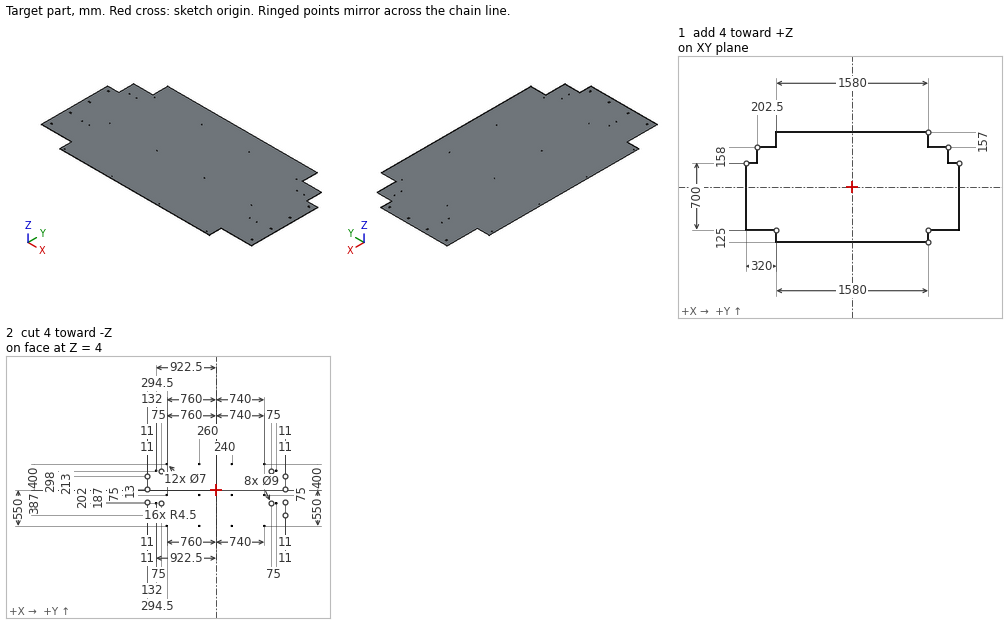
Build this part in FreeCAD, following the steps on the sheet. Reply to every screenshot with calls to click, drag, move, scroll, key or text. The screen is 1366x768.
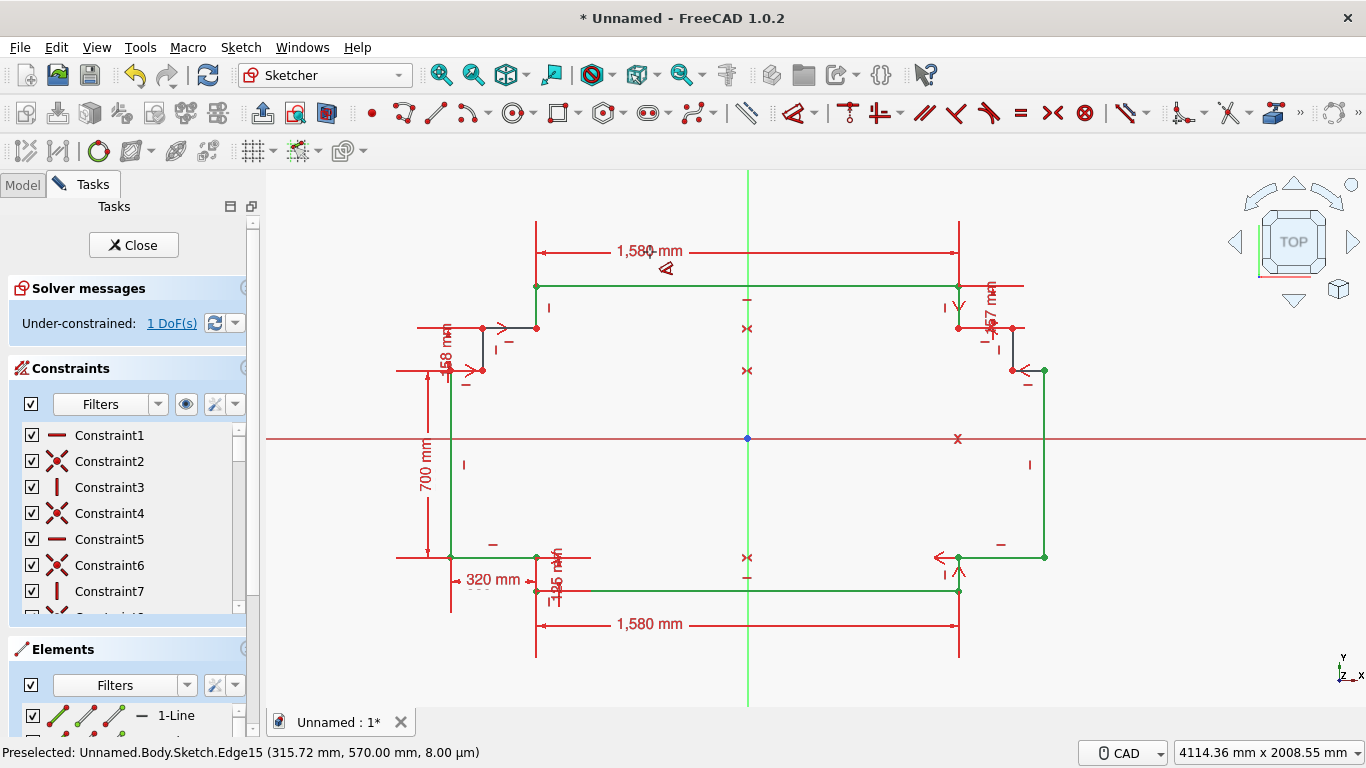
click(520, 328)
click(509, 294)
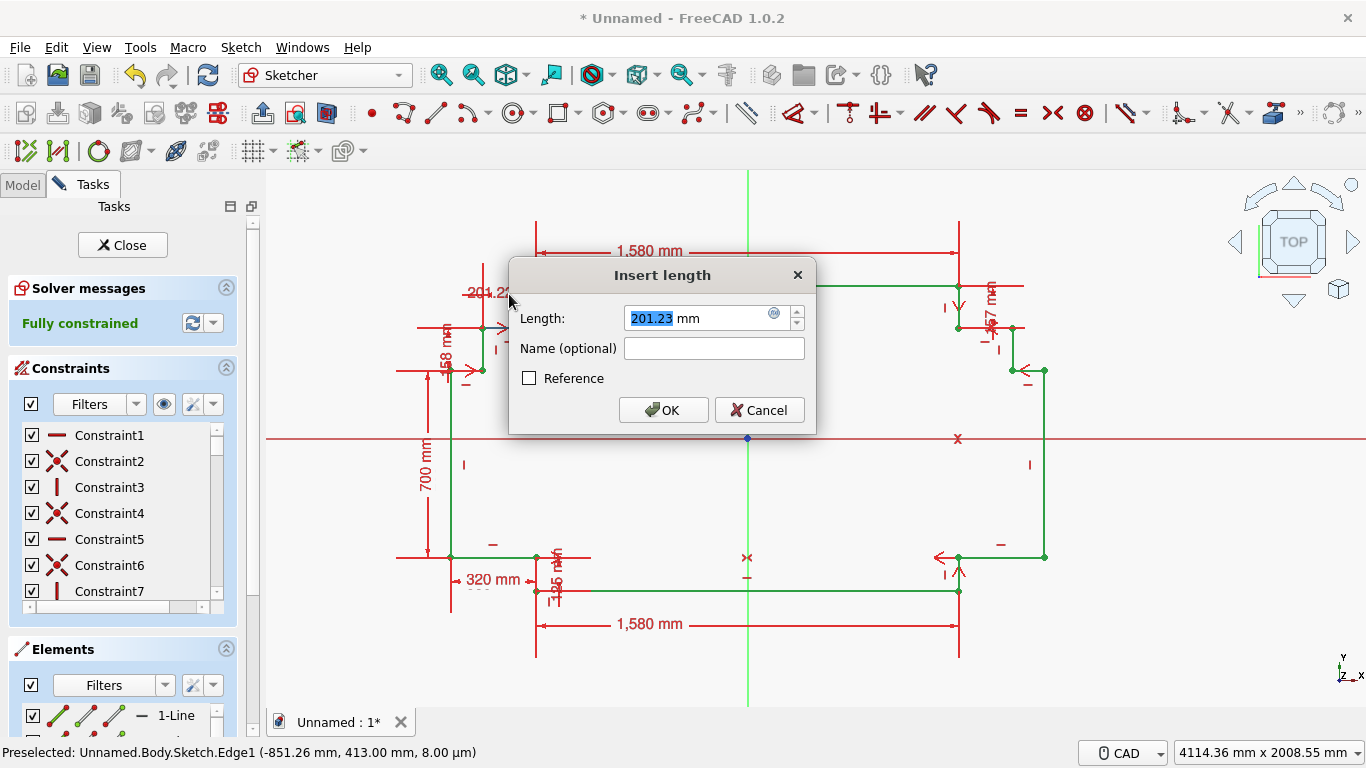
text(202.5)
key(Return)
key(Escape)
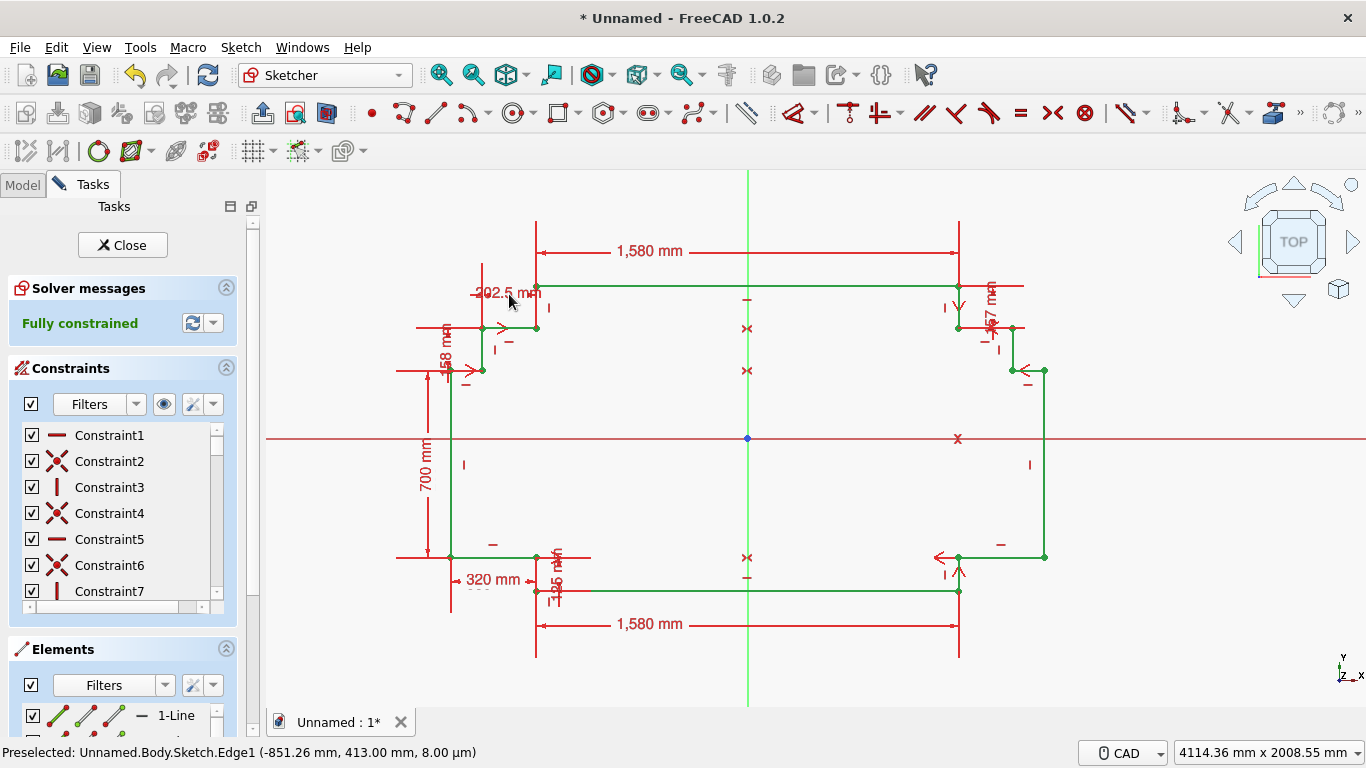
click(123, 245)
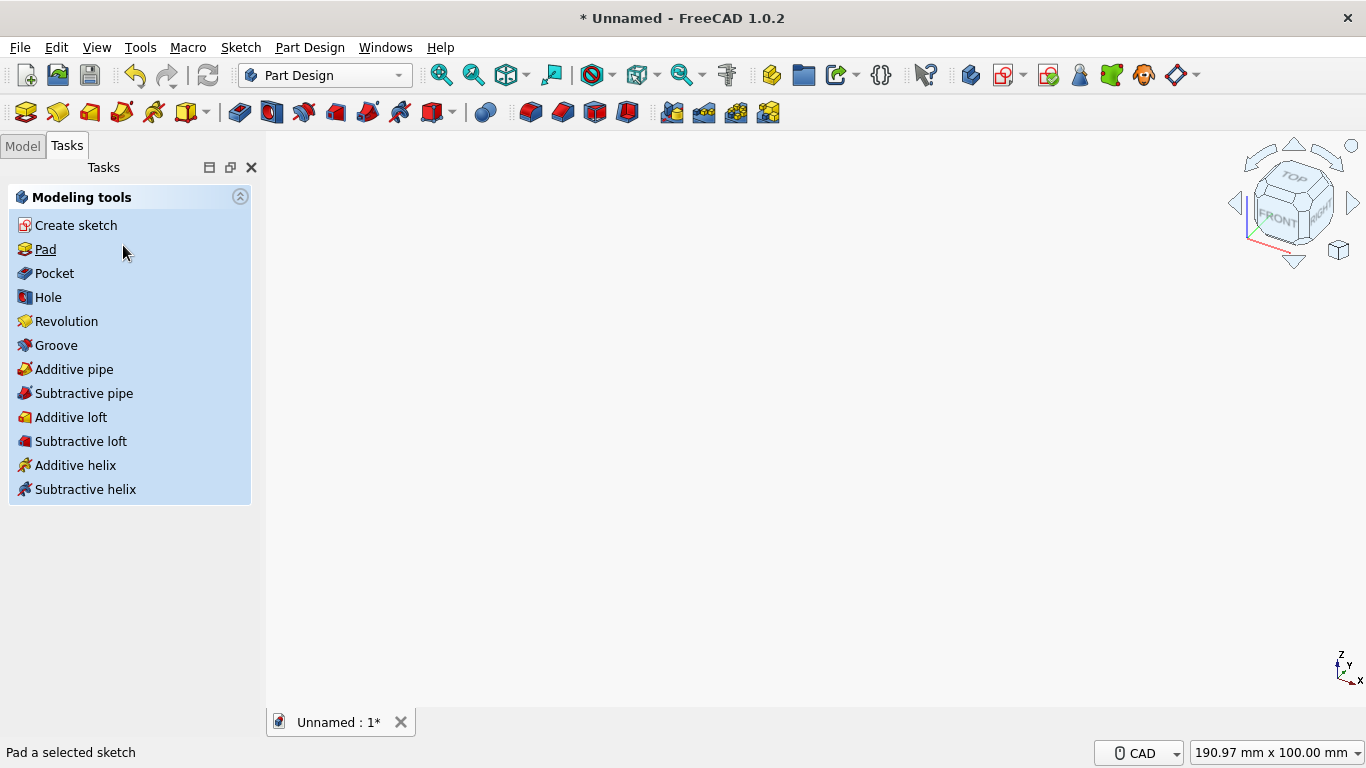
click(26, 112)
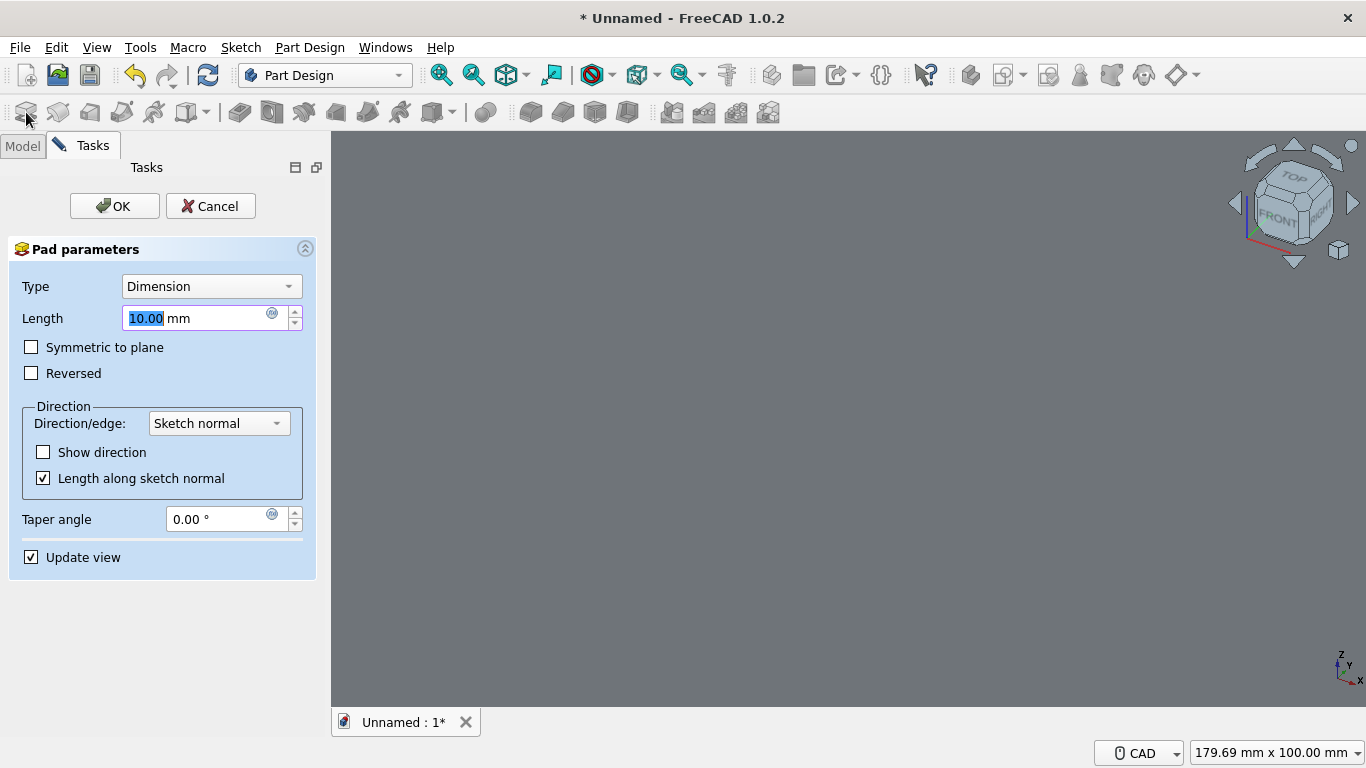
text(4)
key(Tab)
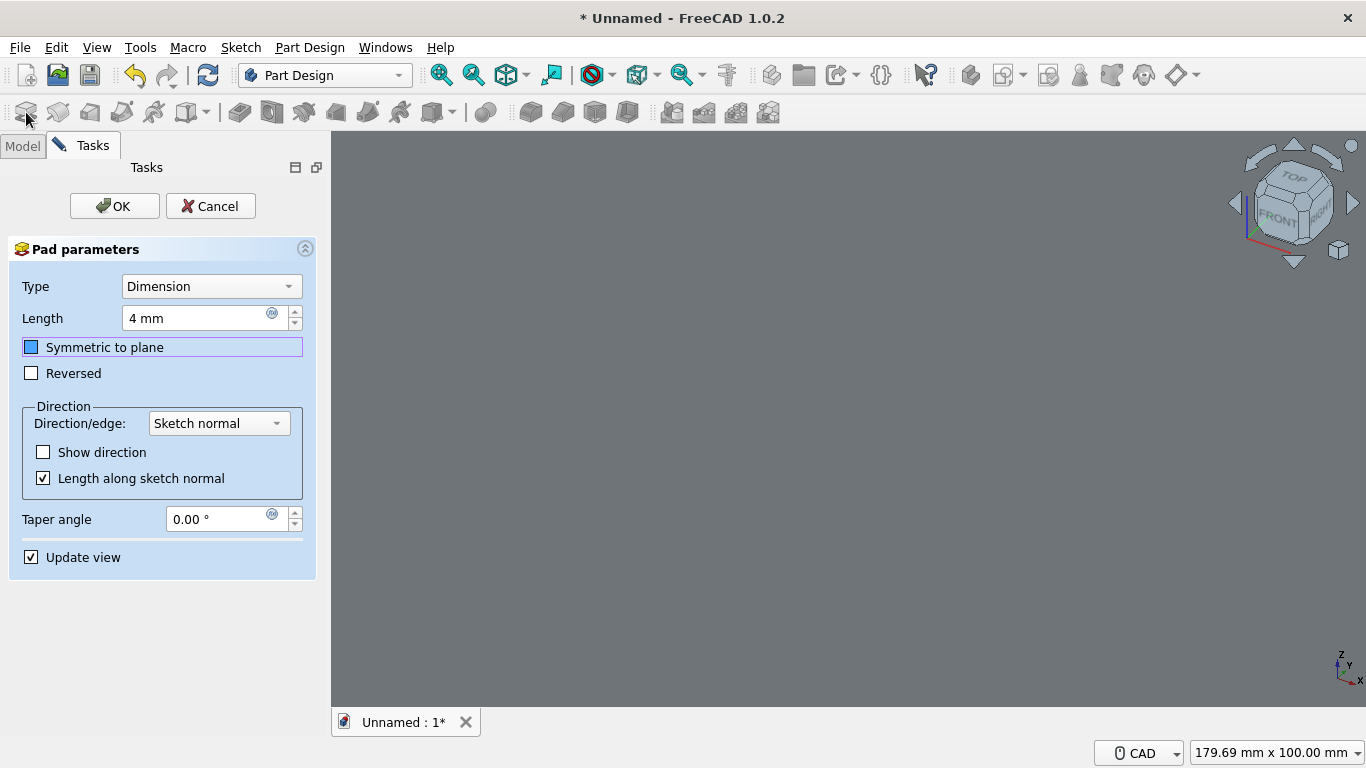
click(115, 206)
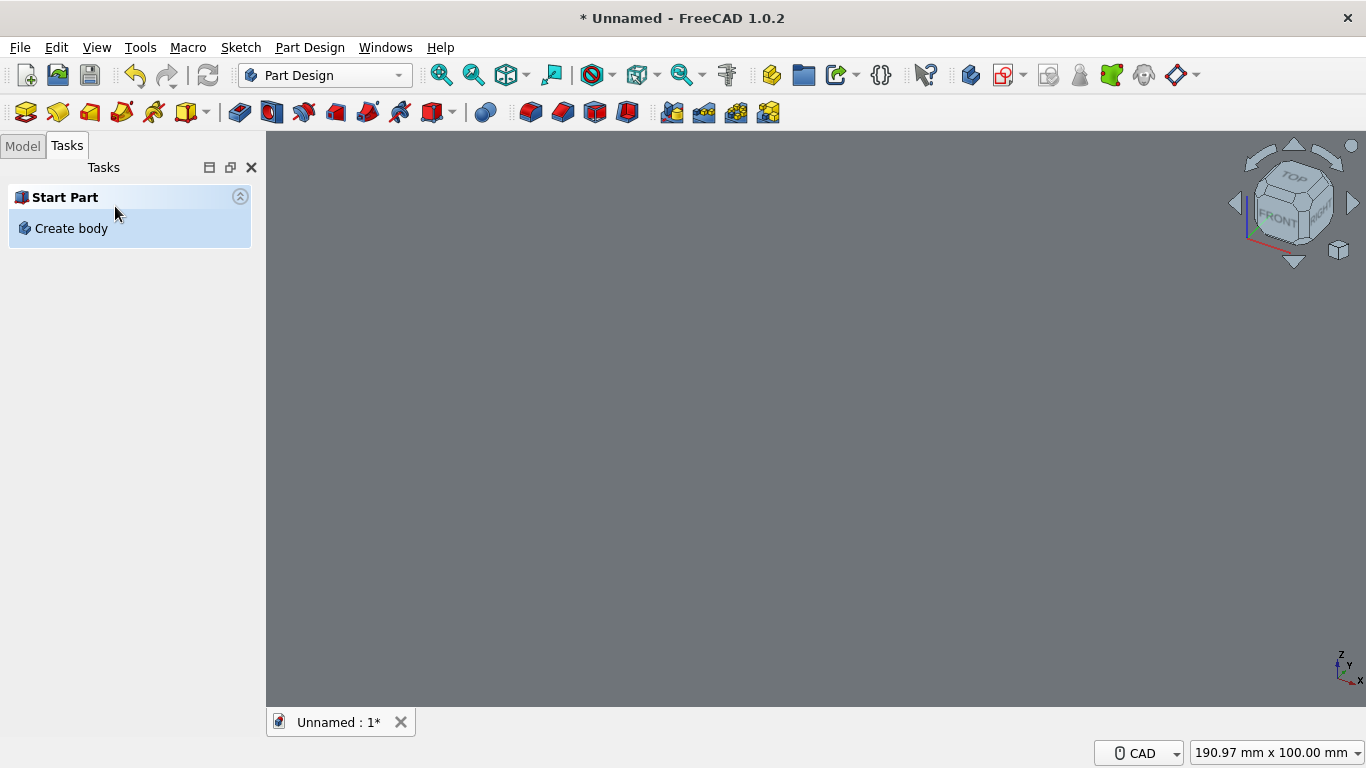
click(442, 76)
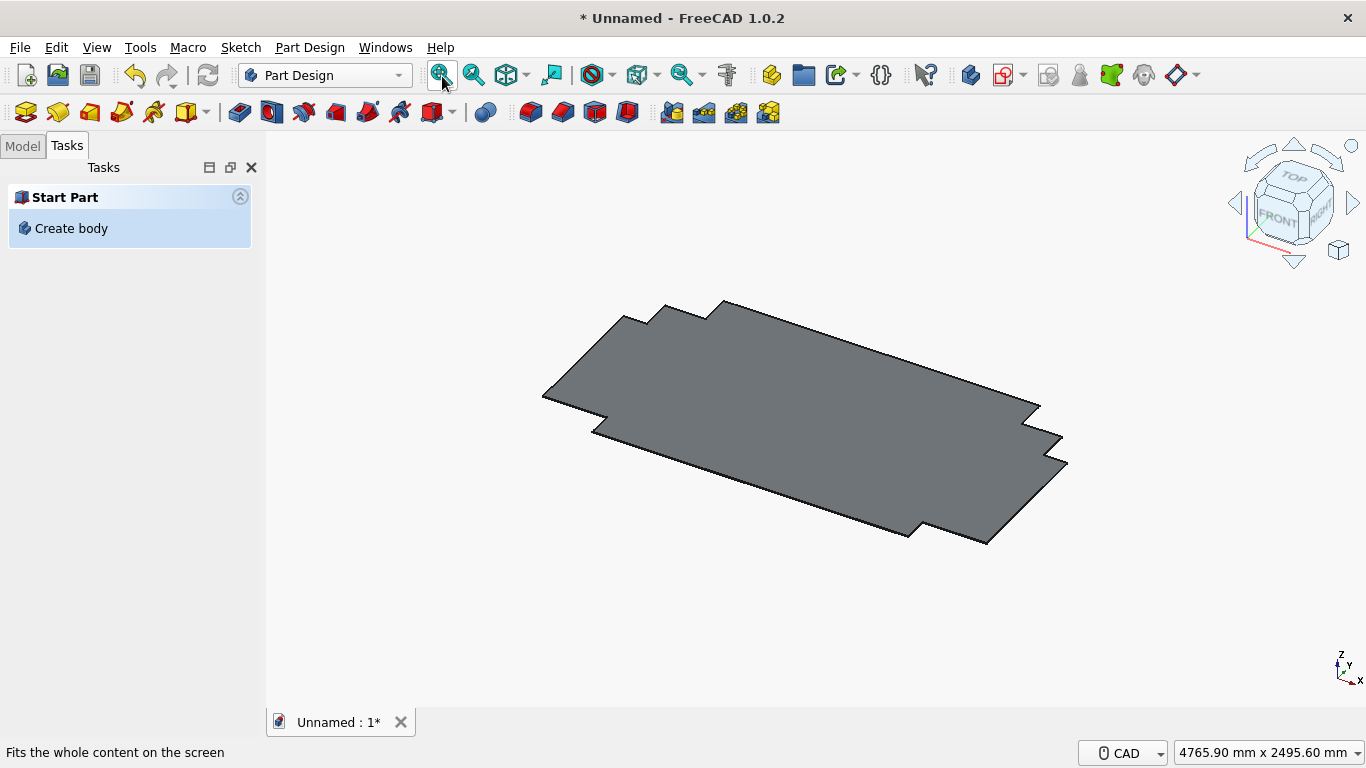
click(879, 439)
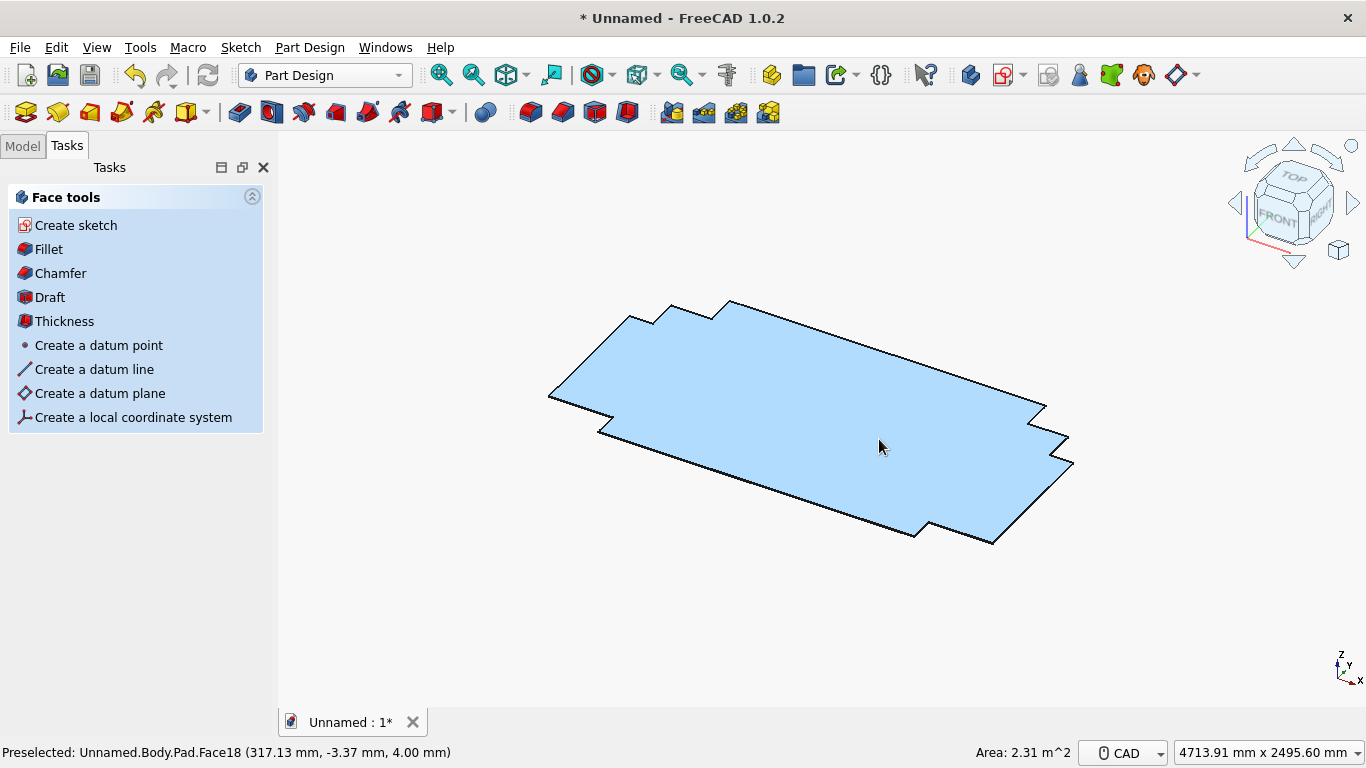
click(1004, 76)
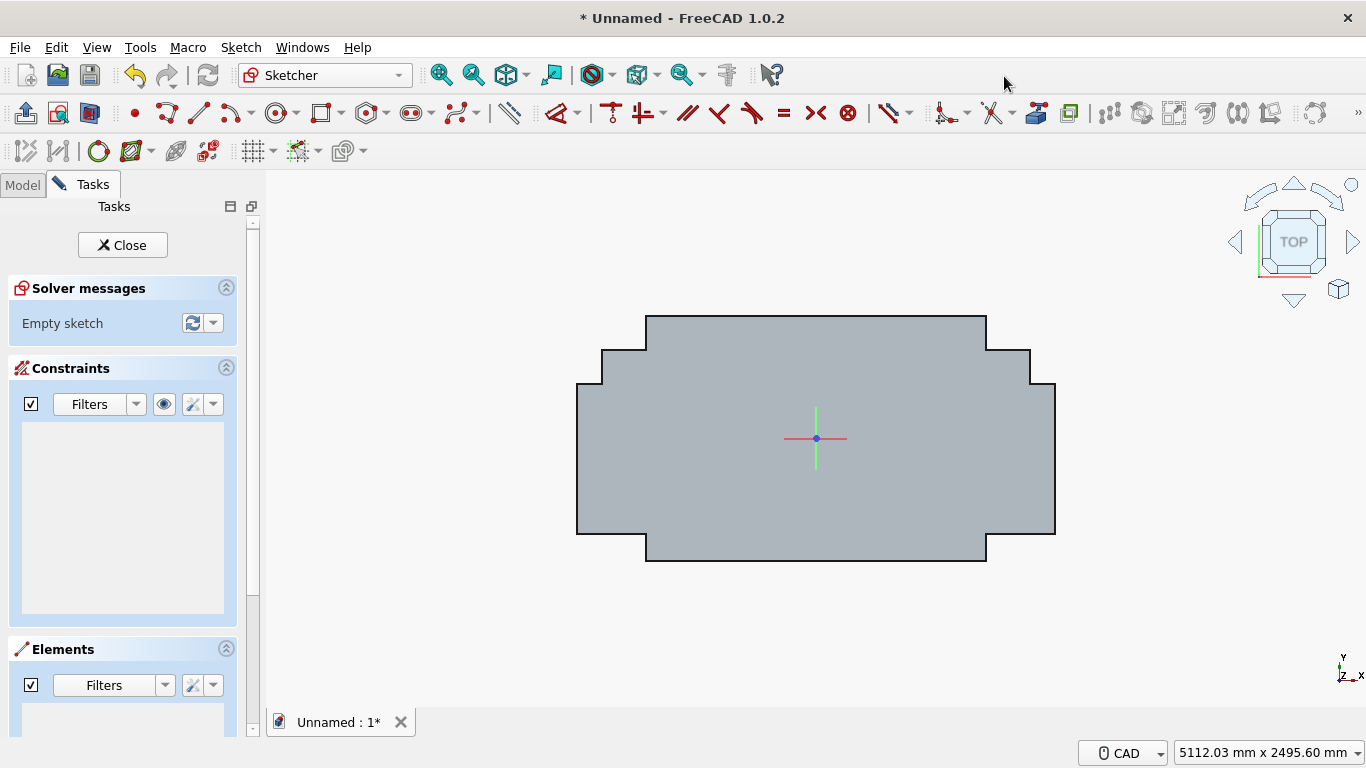
scroll(955, 487, up, 2)